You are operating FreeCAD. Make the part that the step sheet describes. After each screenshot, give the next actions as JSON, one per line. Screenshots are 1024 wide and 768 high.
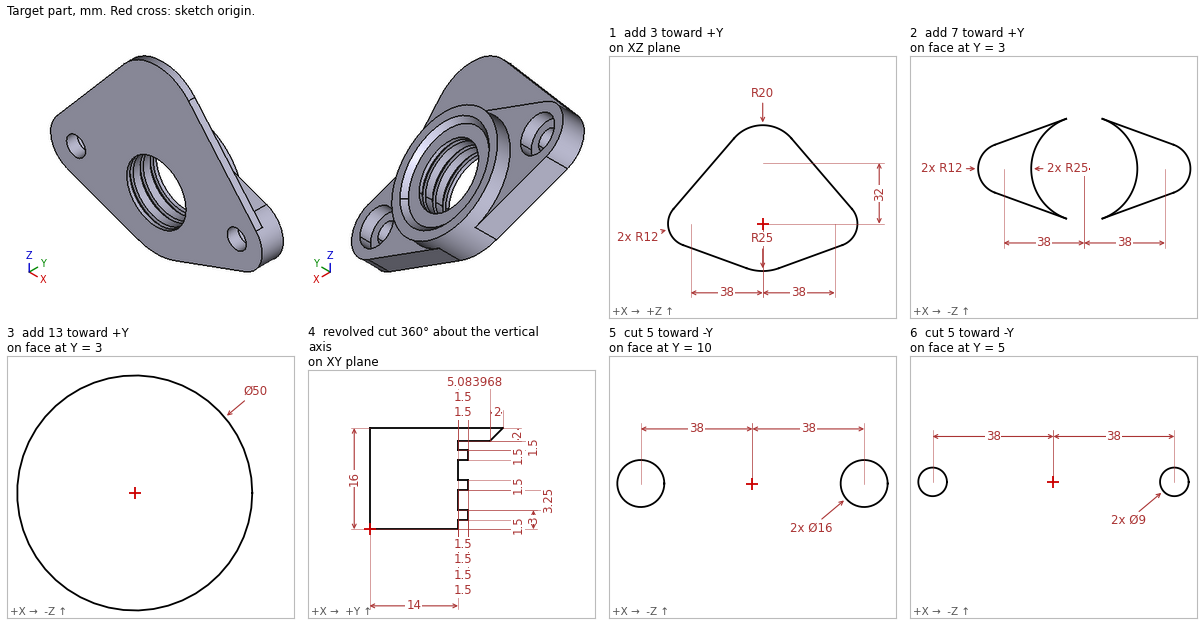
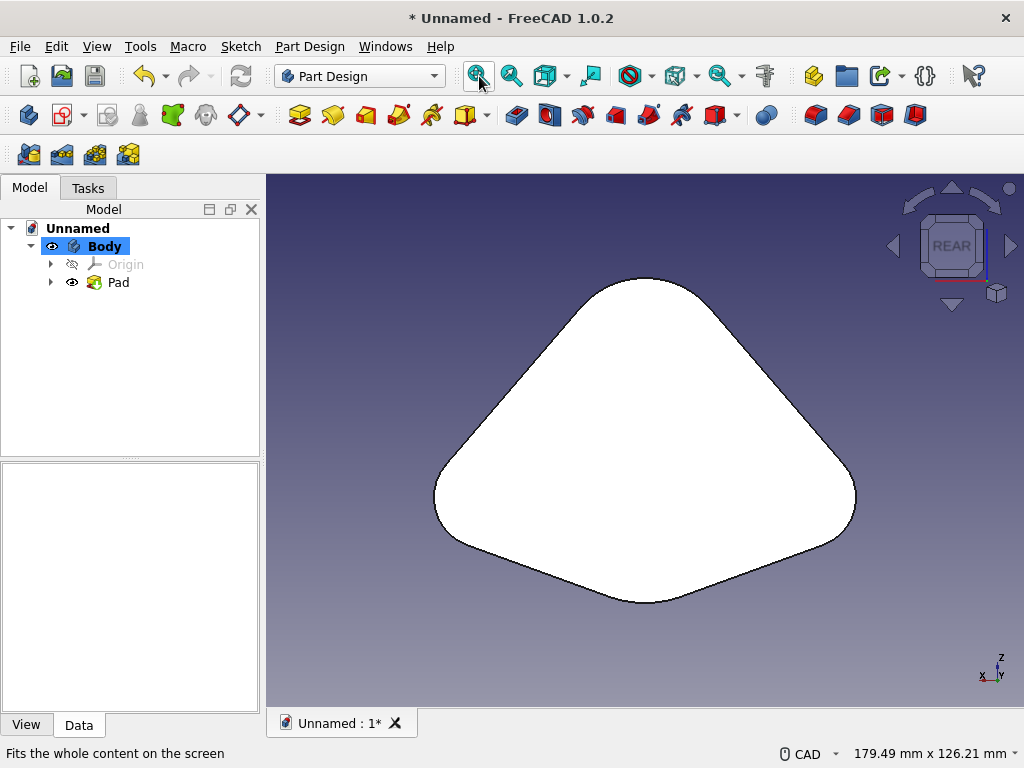
{"action": "left_click", "coordinate": [645, 439]}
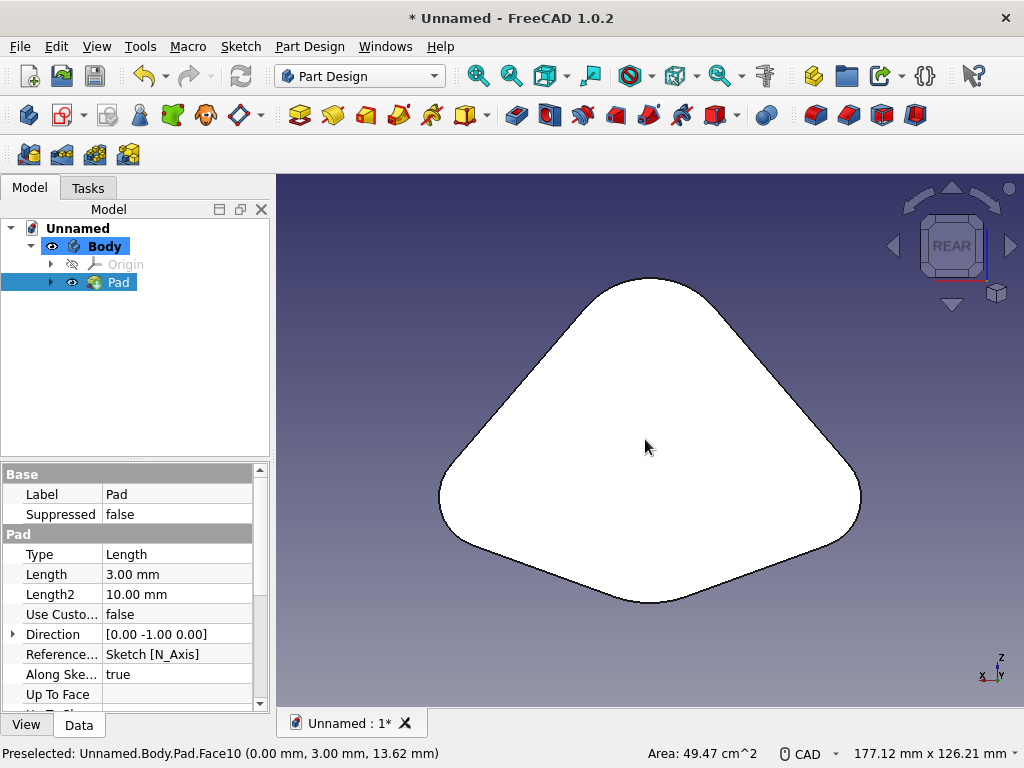
{"action": "left_click", "coordinate": [62, 116]}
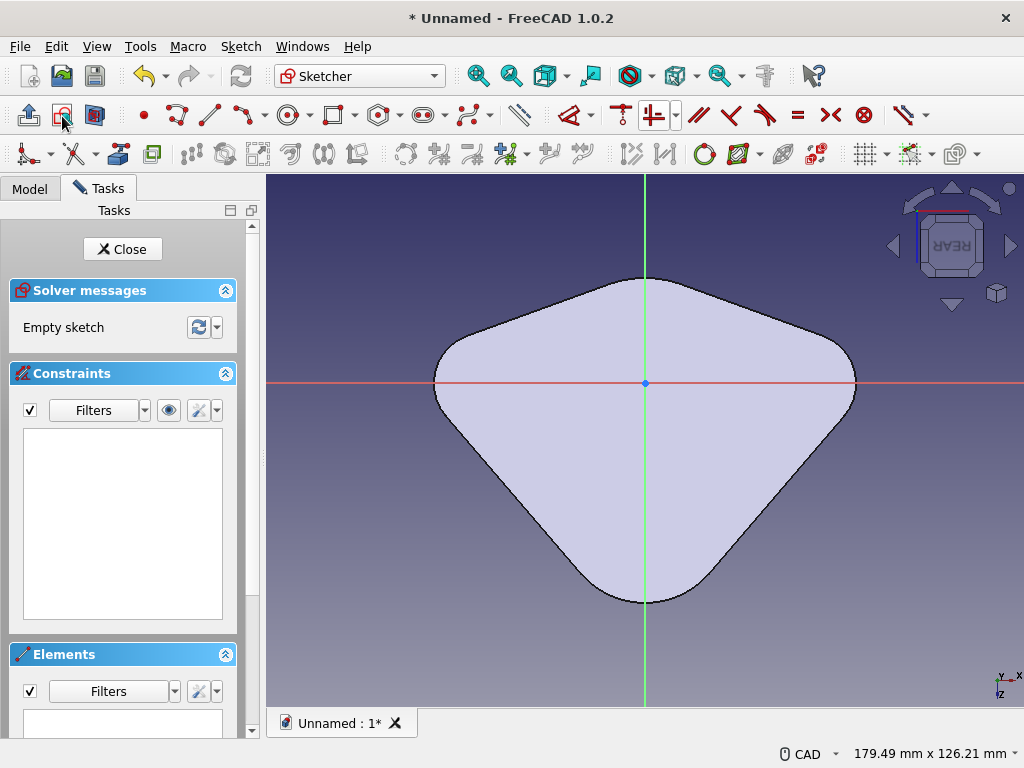
{"action": "scroll", "coordinate": [294, 679], "scroll_direction": "down", "scroll_amount": 1}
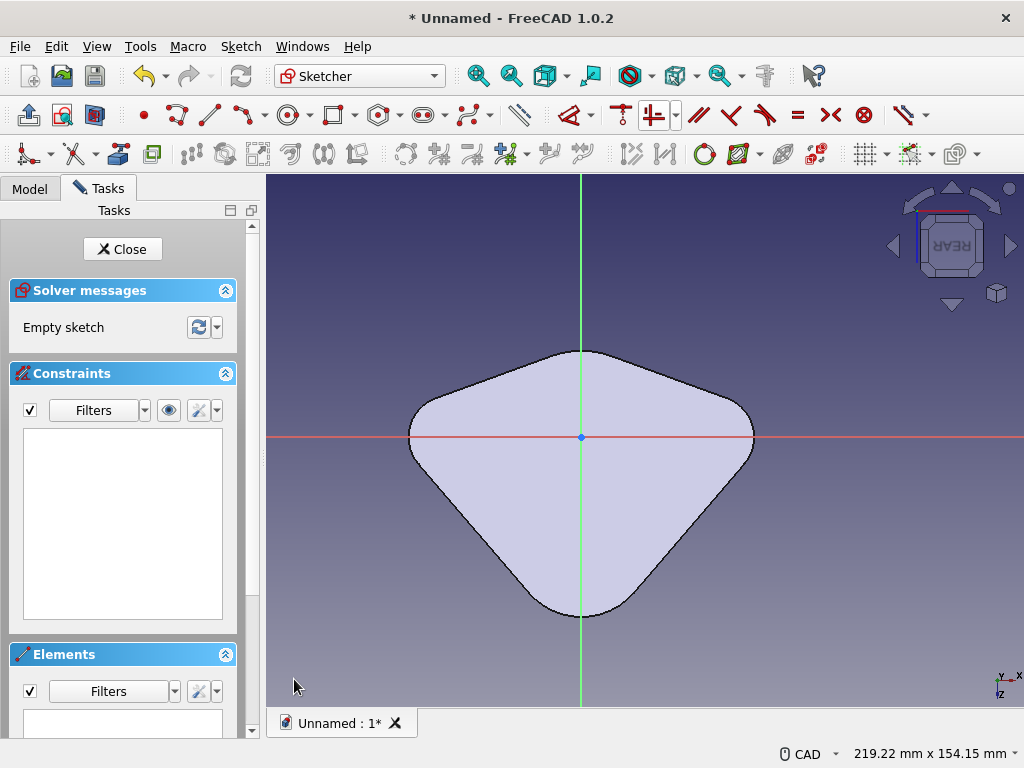
{"action": "left_click", "coordinate": [210, 116]}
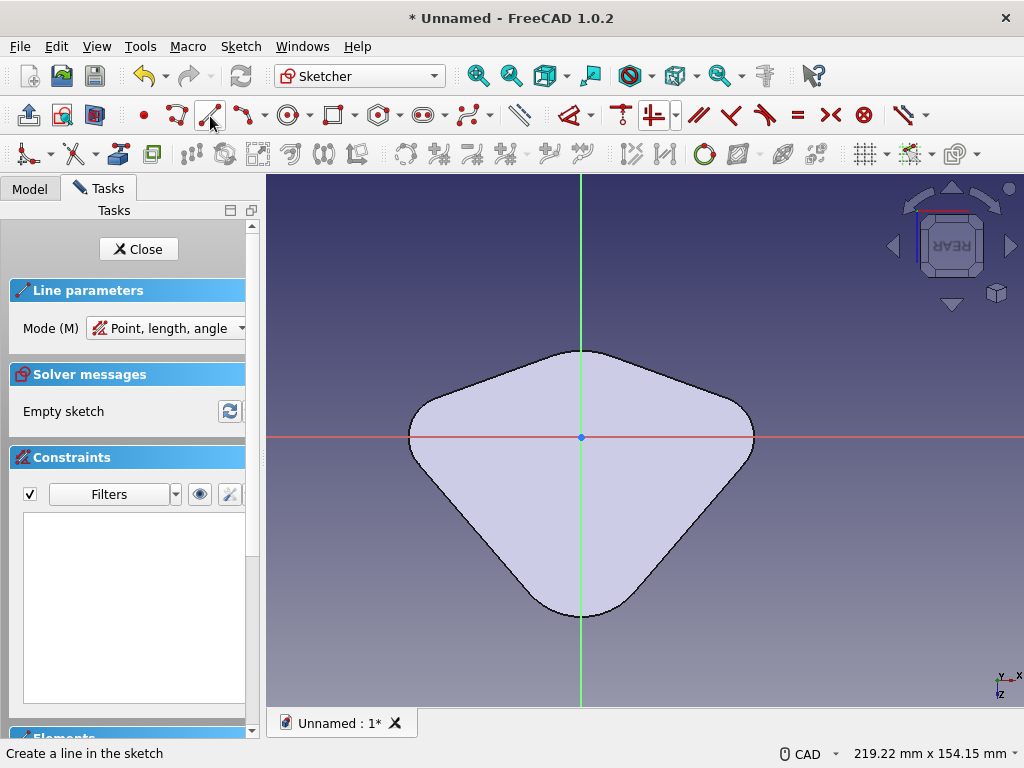
{"action": "left_click", "coordinate": [436, 476]}
{"action": "left_click", "coordinate": [552, 518]}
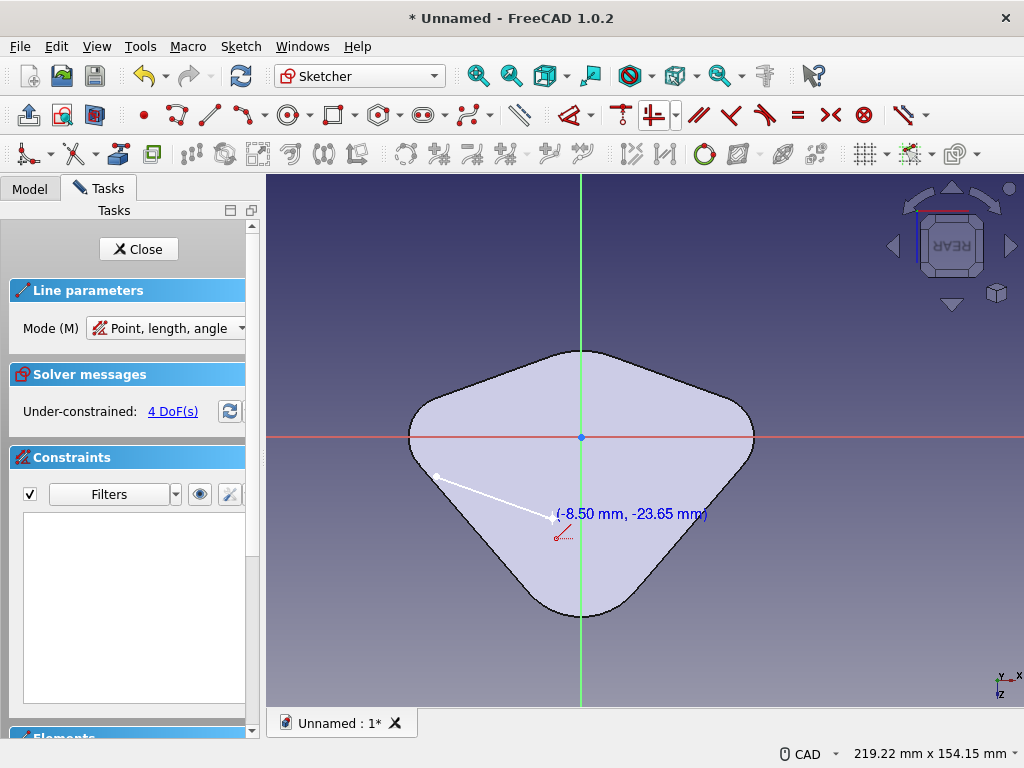
{"action": "left_click", "coordinate": [552, 356]}
{"action": "left_click", "coordinate": [436, 398]}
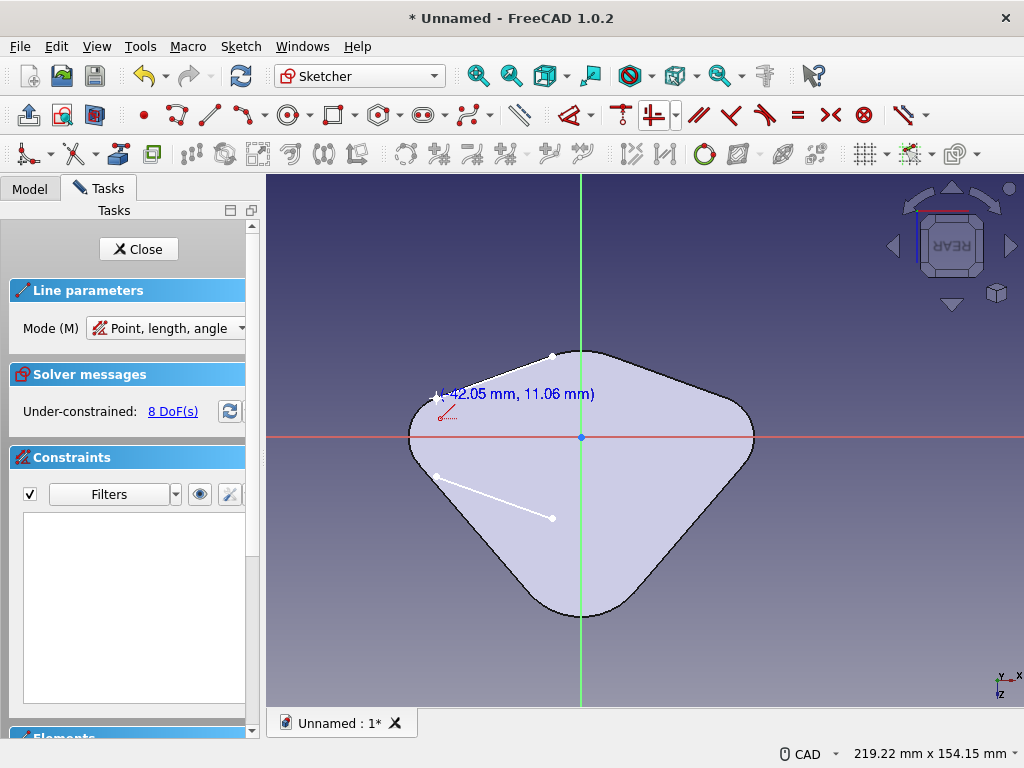
{"action": "left_click", "coordinate": [242, 116]}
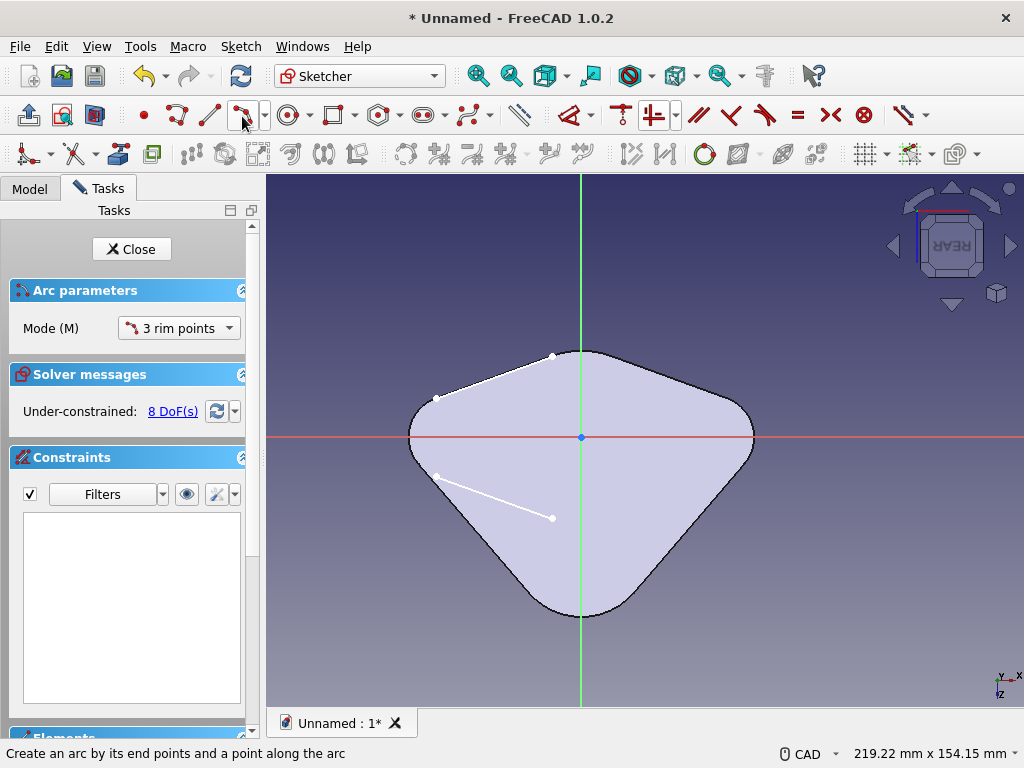
{"action": "left_click", "coordinate": [552, 519]}
{"action": "left_click", "coordinate": [552, 357]}
{"action": "left_click", "coordinate": [498, 416]}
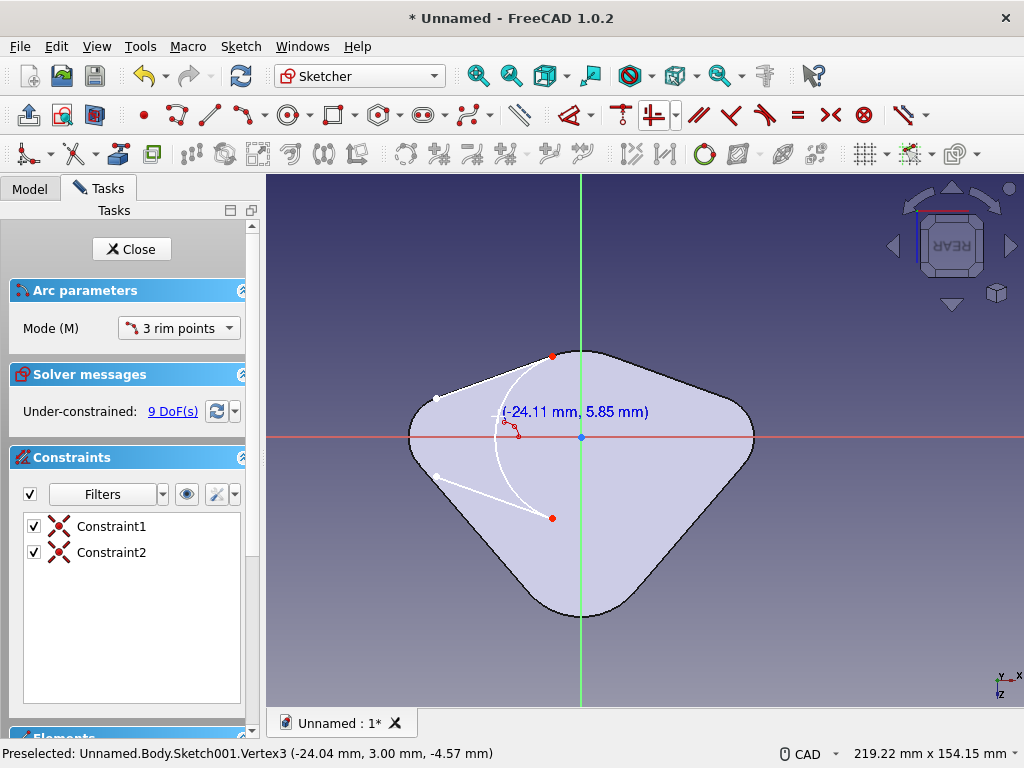
{"action": "left_click", "coordinate": [436, 399]}
{"action": "left_click", "coordinate": [436, 477]}
{"action": "left_click", "coordinate": [413, 418]}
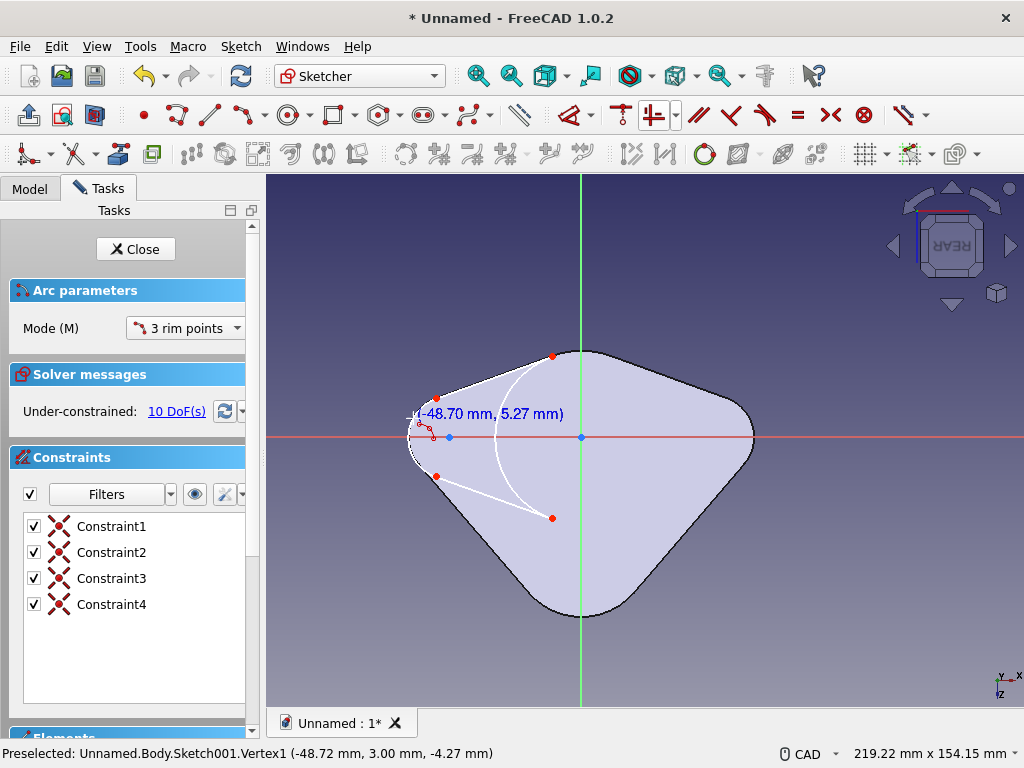
{"action": "left_click", "coordinate": [210, 116]}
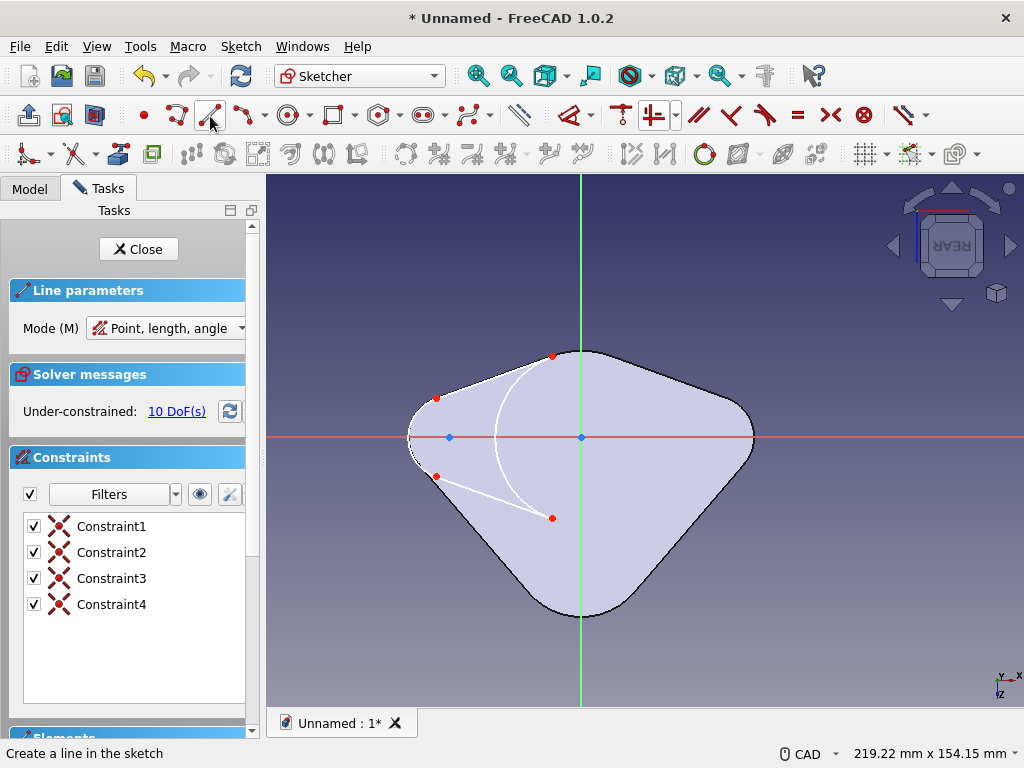
{"action": "left_click", "coordinate": [611, 518]}
{"action": "left_click", "coordinate": [727, 476]}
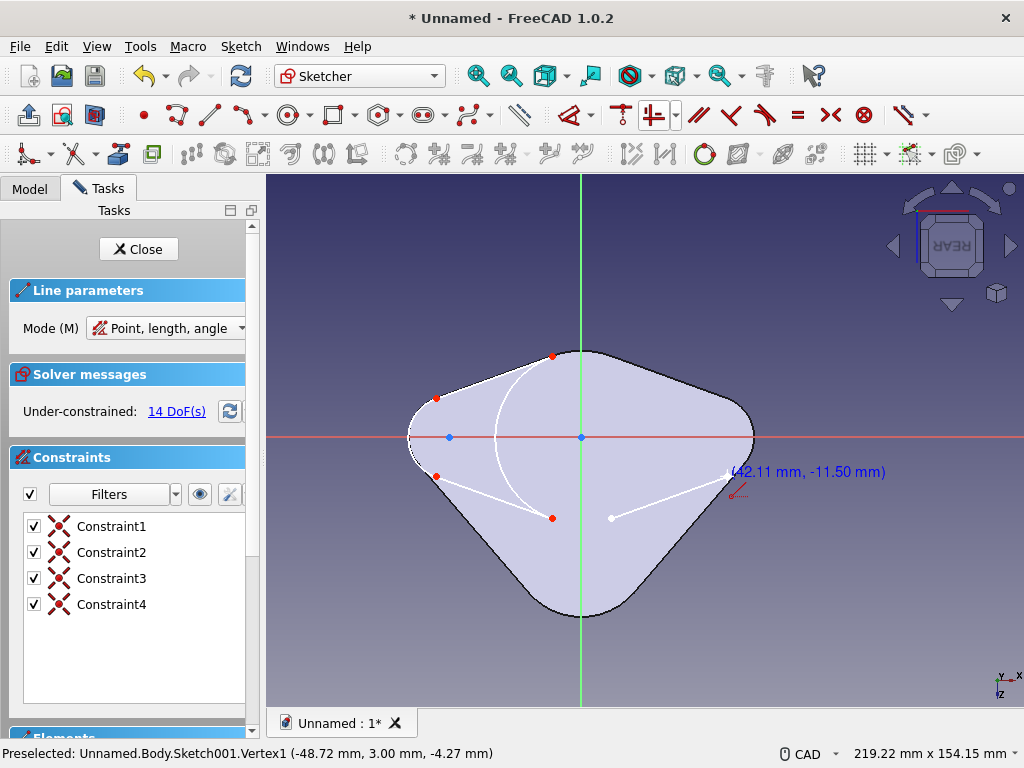
{"action": "left_click", "coordinate": [727, 398]}
{"action": "left_click", "coordinate": [611, 356]}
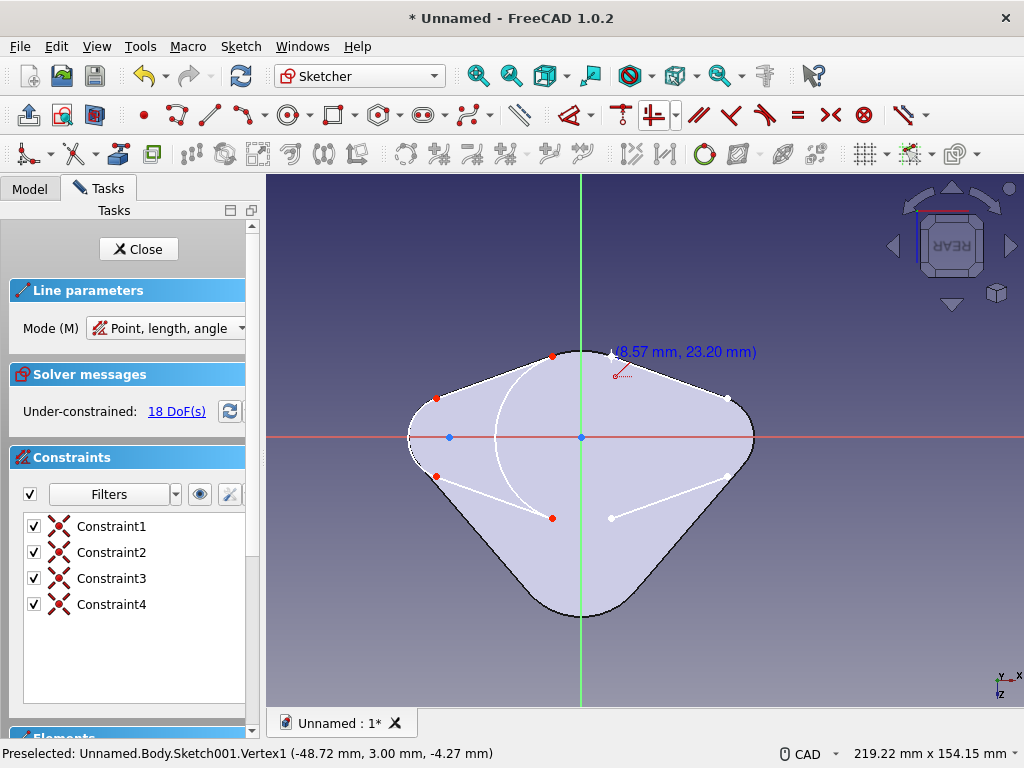
{"action": "left_click", "coordinate": [242, 116]}